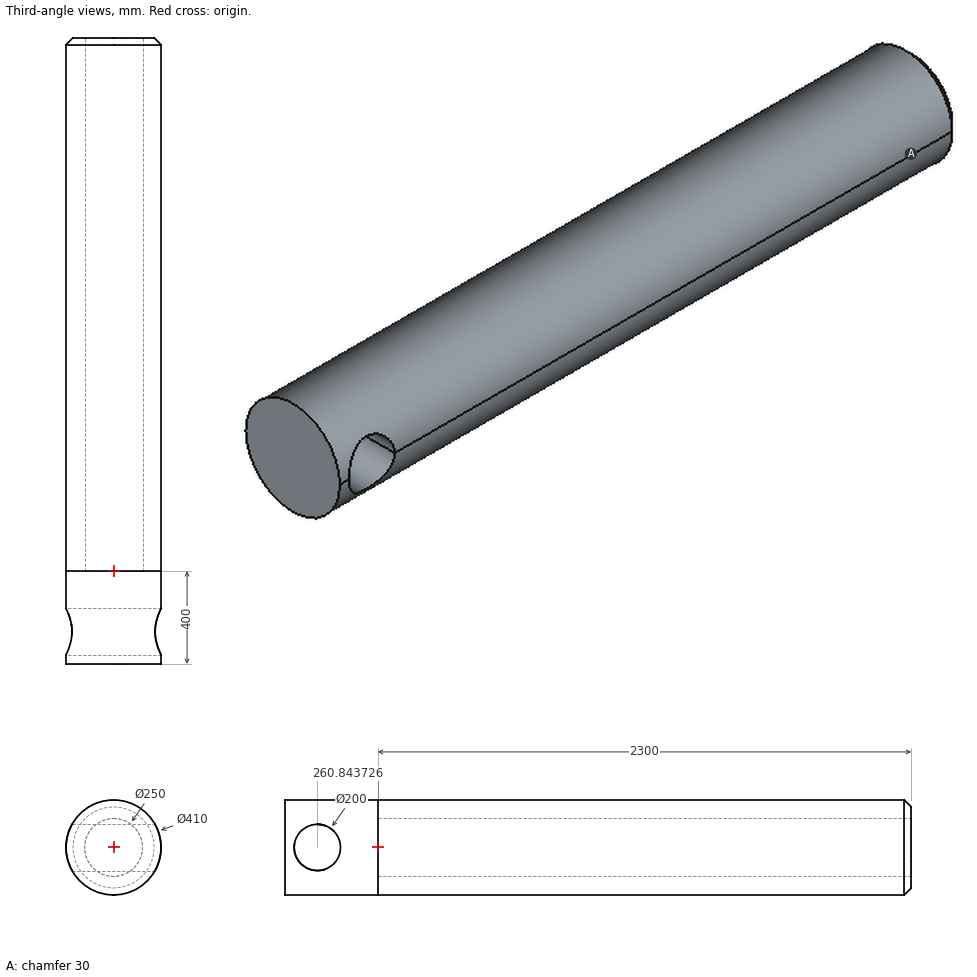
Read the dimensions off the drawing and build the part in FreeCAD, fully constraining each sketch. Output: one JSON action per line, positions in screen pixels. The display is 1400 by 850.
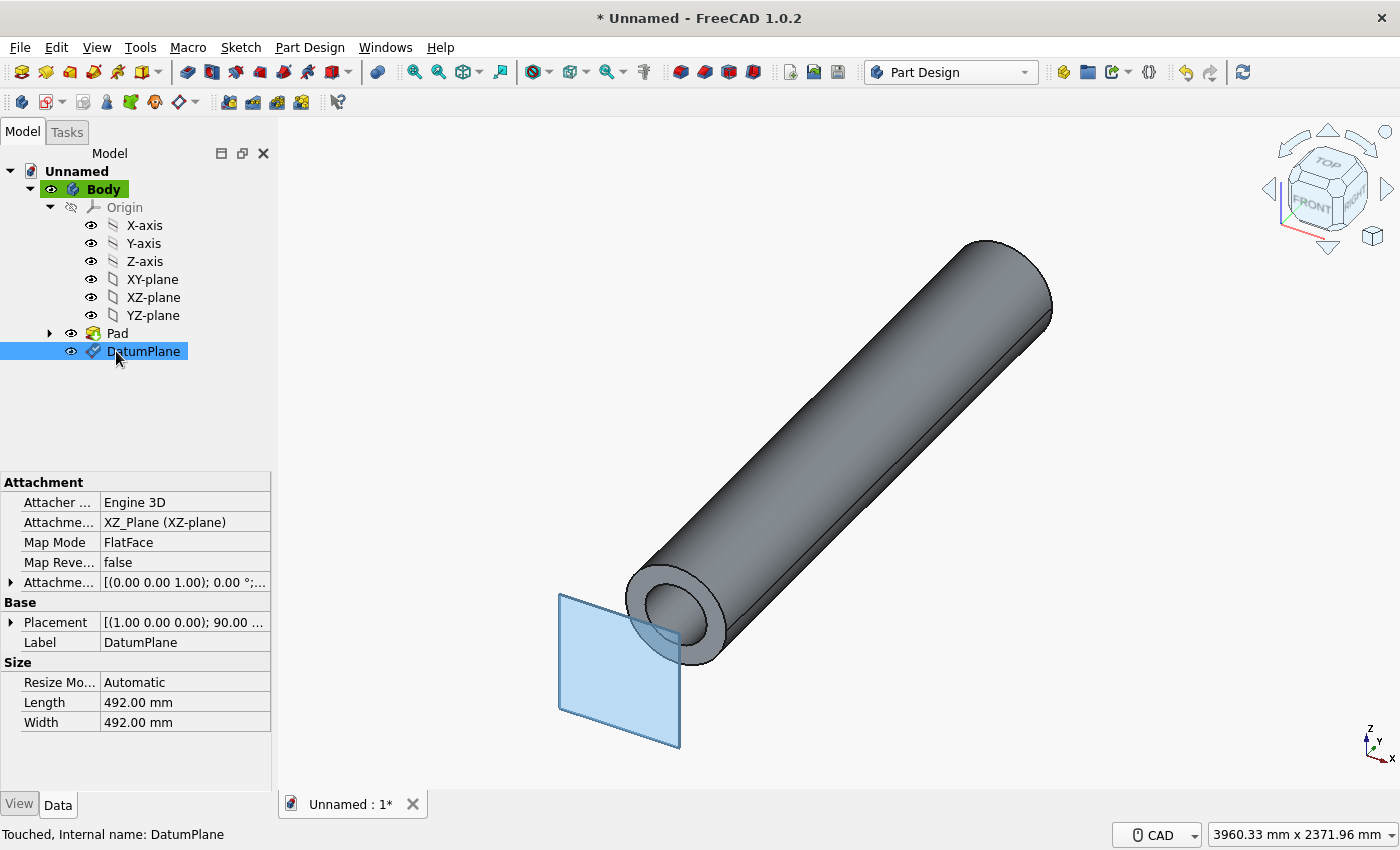
{"action": "left_click", "coordinate": [46, 102]}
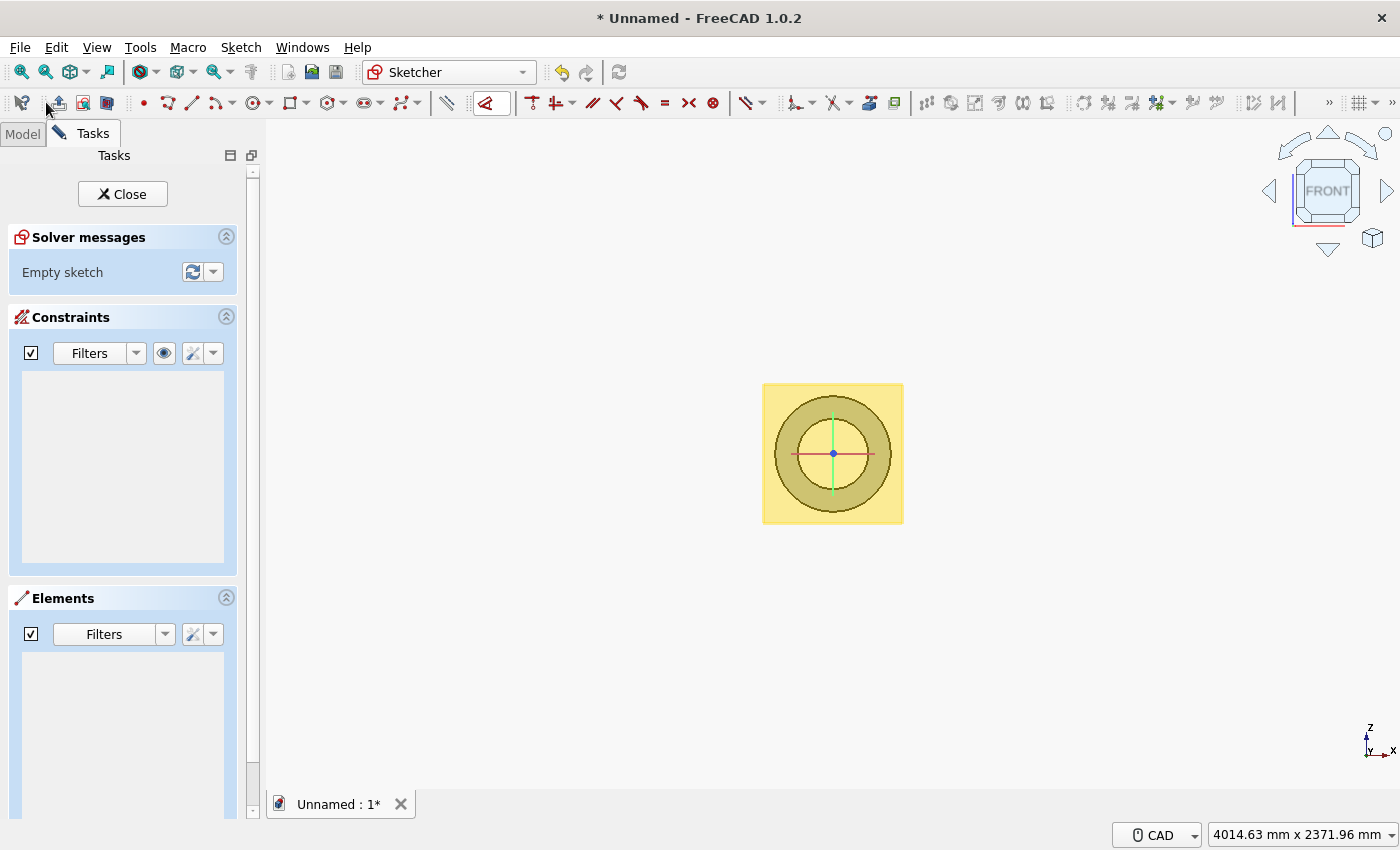
{"action": "scroll", "coordinate": [855, 454], "scroll_direction": "up", "scroll_amount": 7}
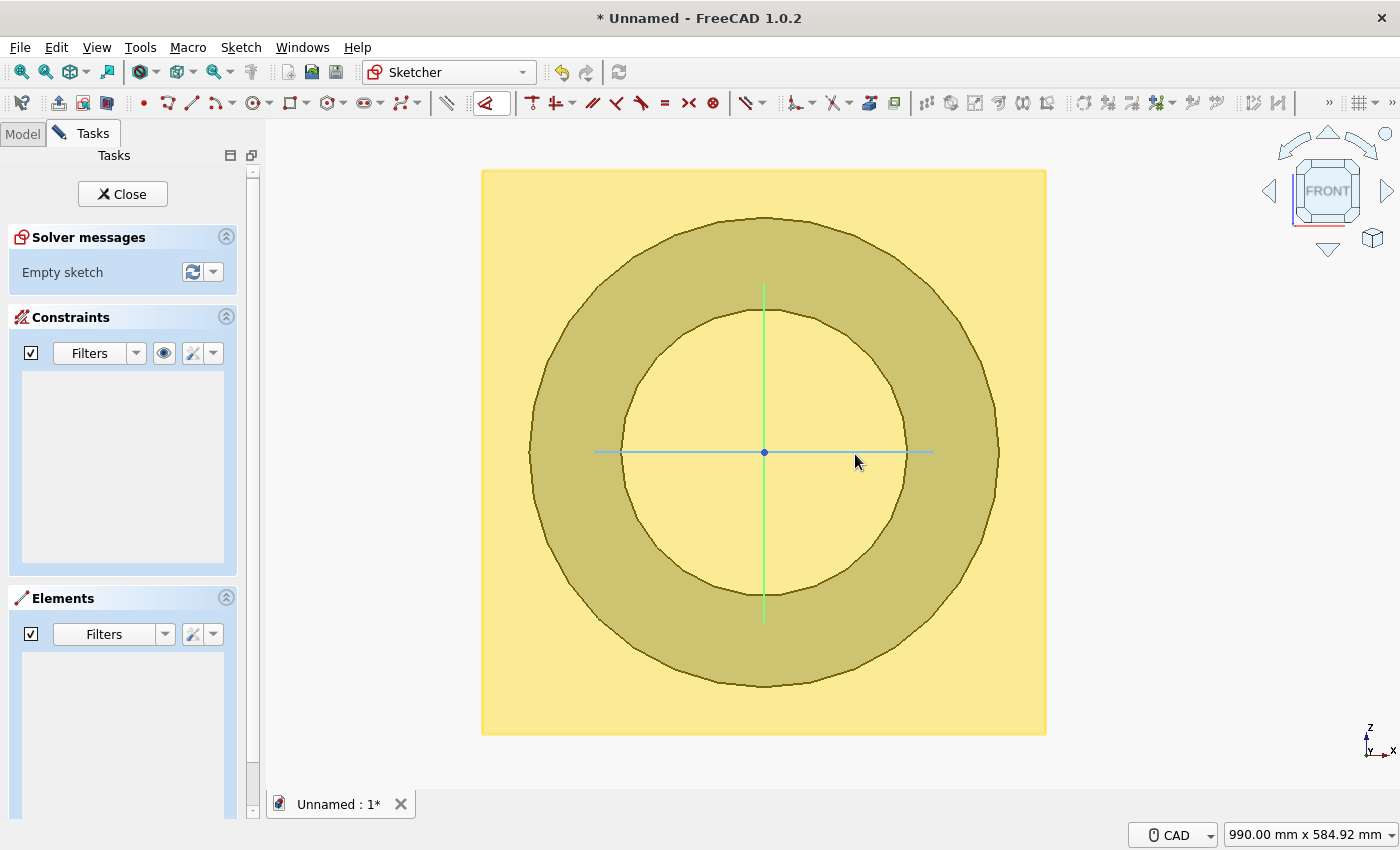
{"action": "left_click", "coordinate": [254, 104]}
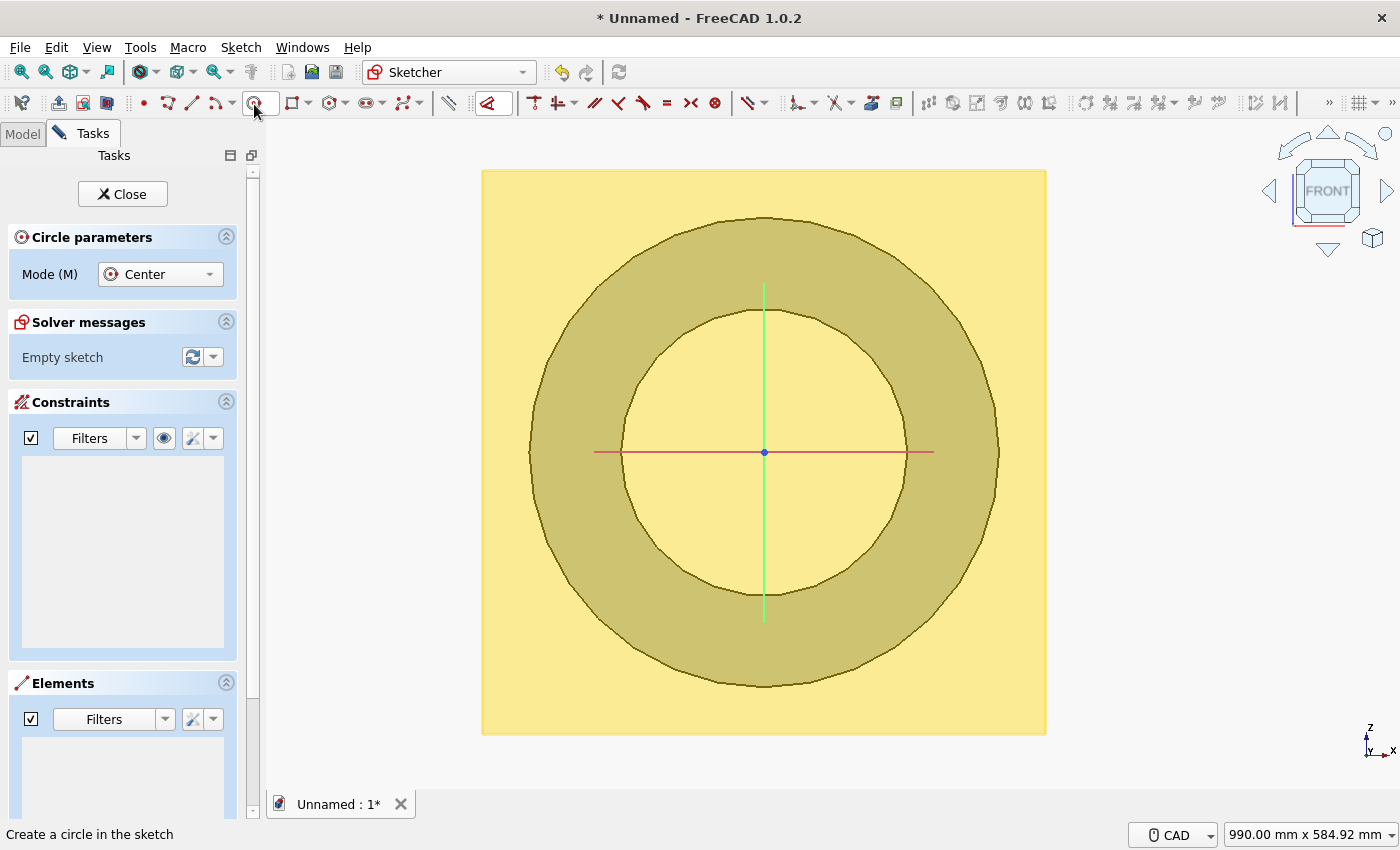
{"action": "left_click", "coordinate": [764, 452]}
{"action": "mouse_move", "coordinate": [930, 286]}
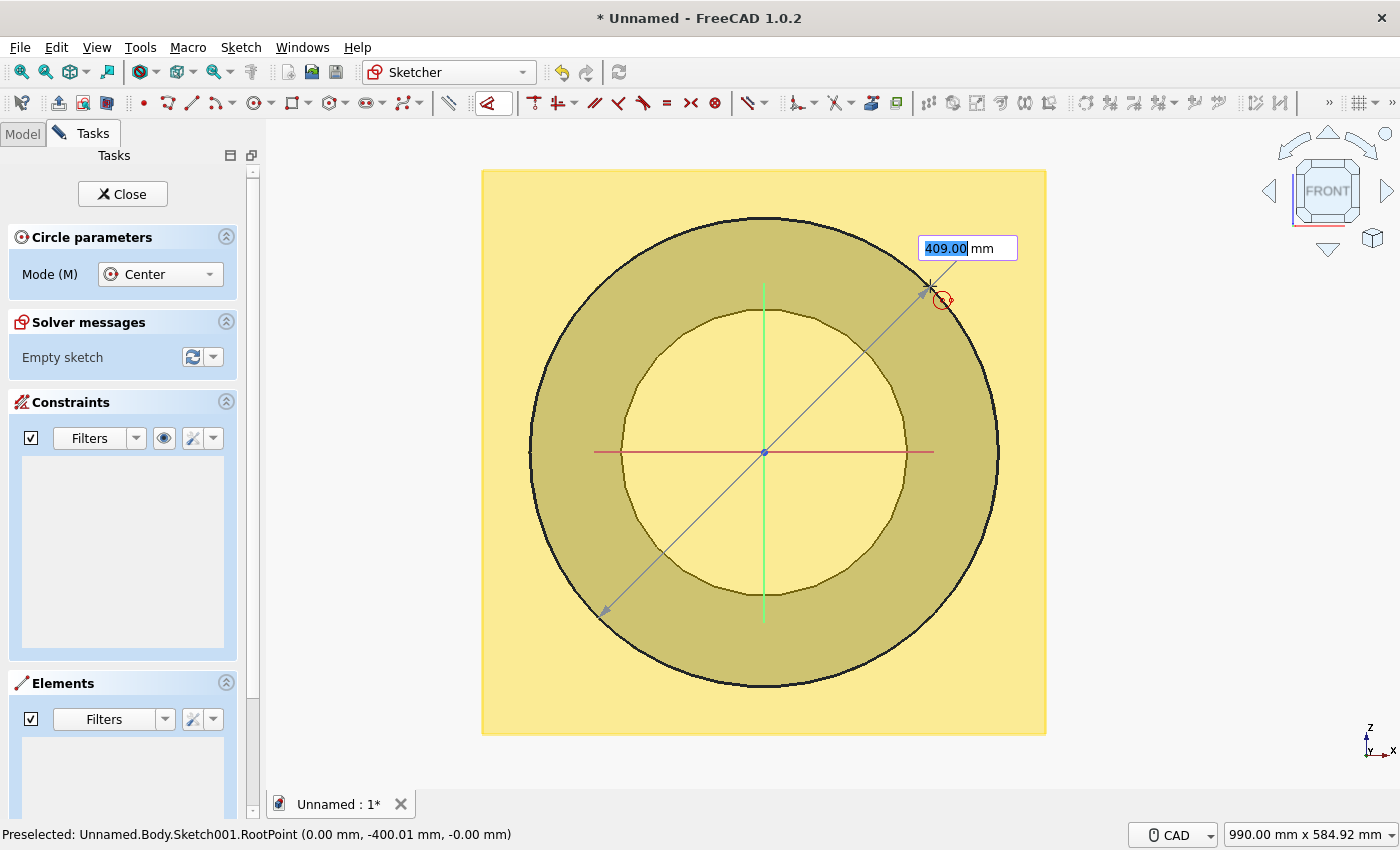
{"action": "type", "text": "410"}
{"action": "key", "text": "Return"}
{"action": "key", "text": "Escape"}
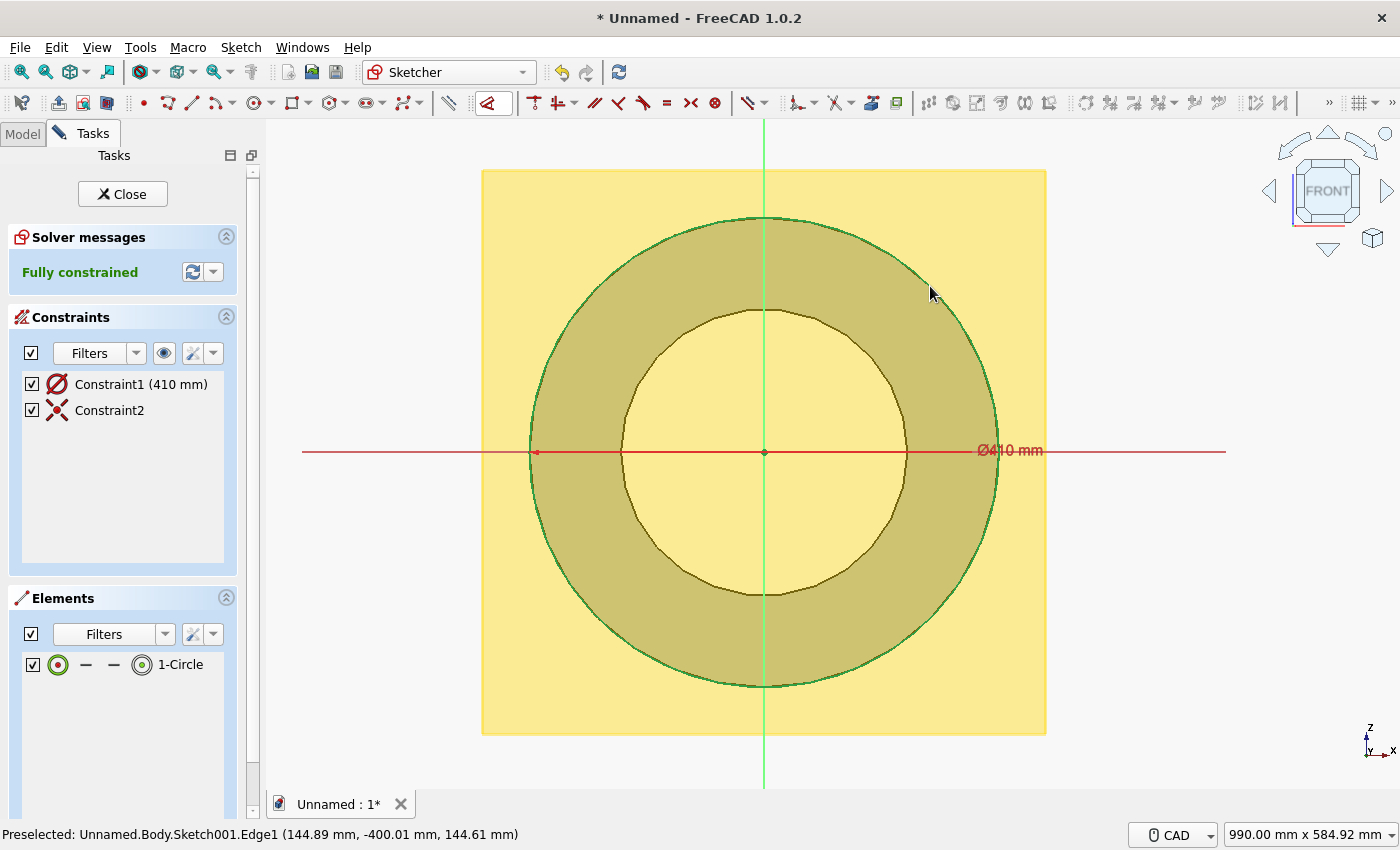
{"action": "left_click", "coordinate": [123, 194]}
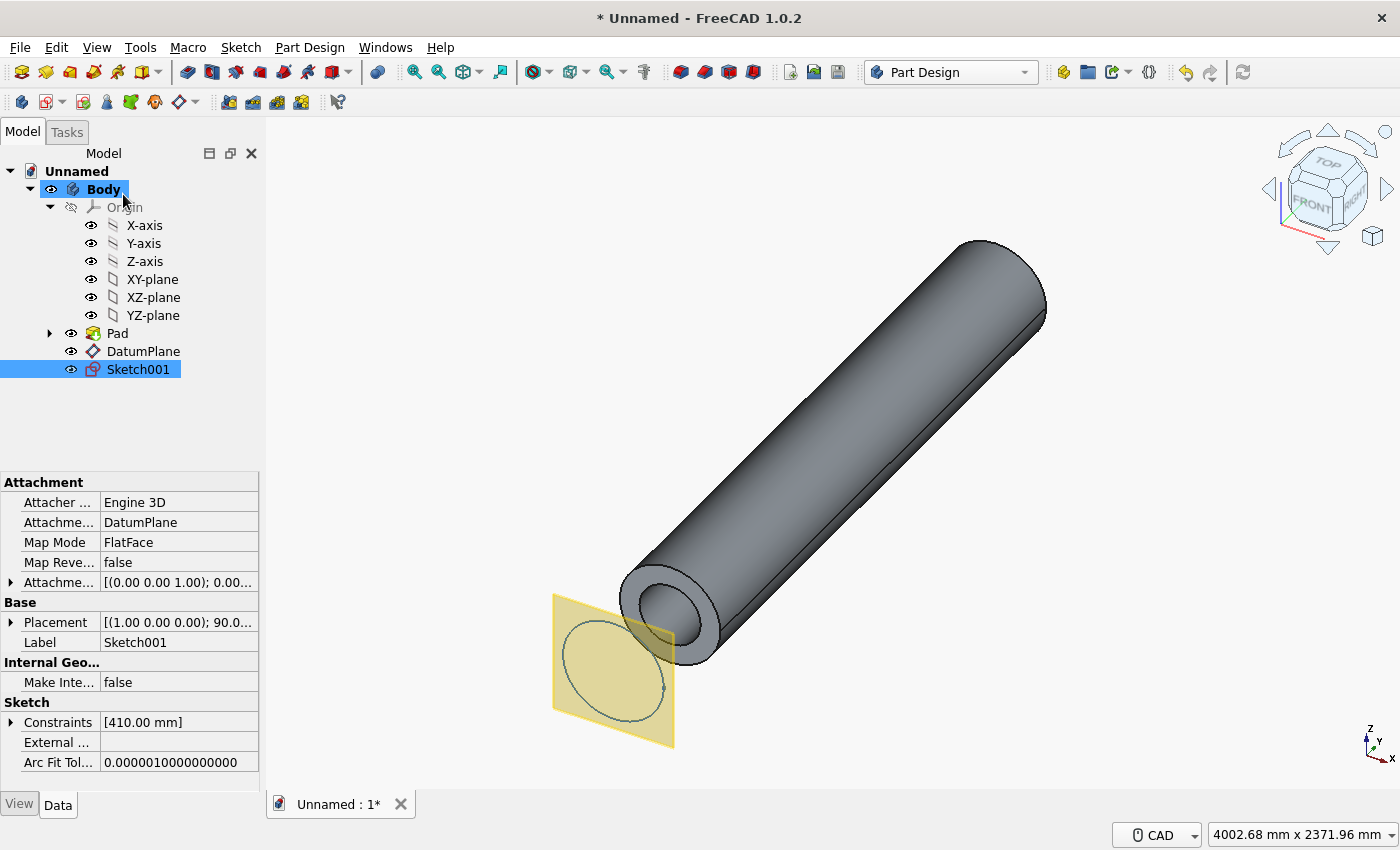
{"action": "left_click", "coordinate": [22, 72]}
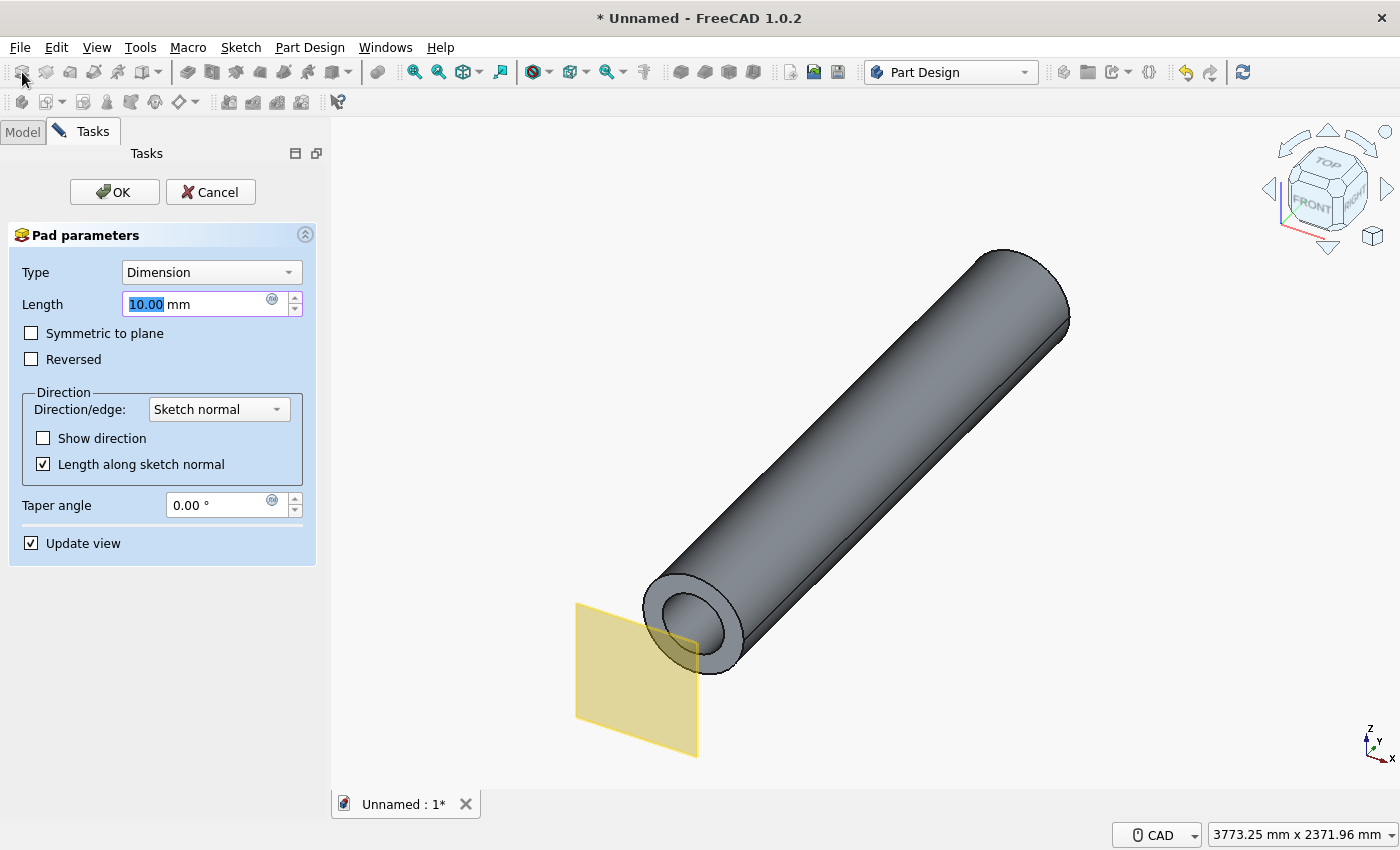
{"action": "type", "text": "400"}
{"action": "key", "text": "Tab"}